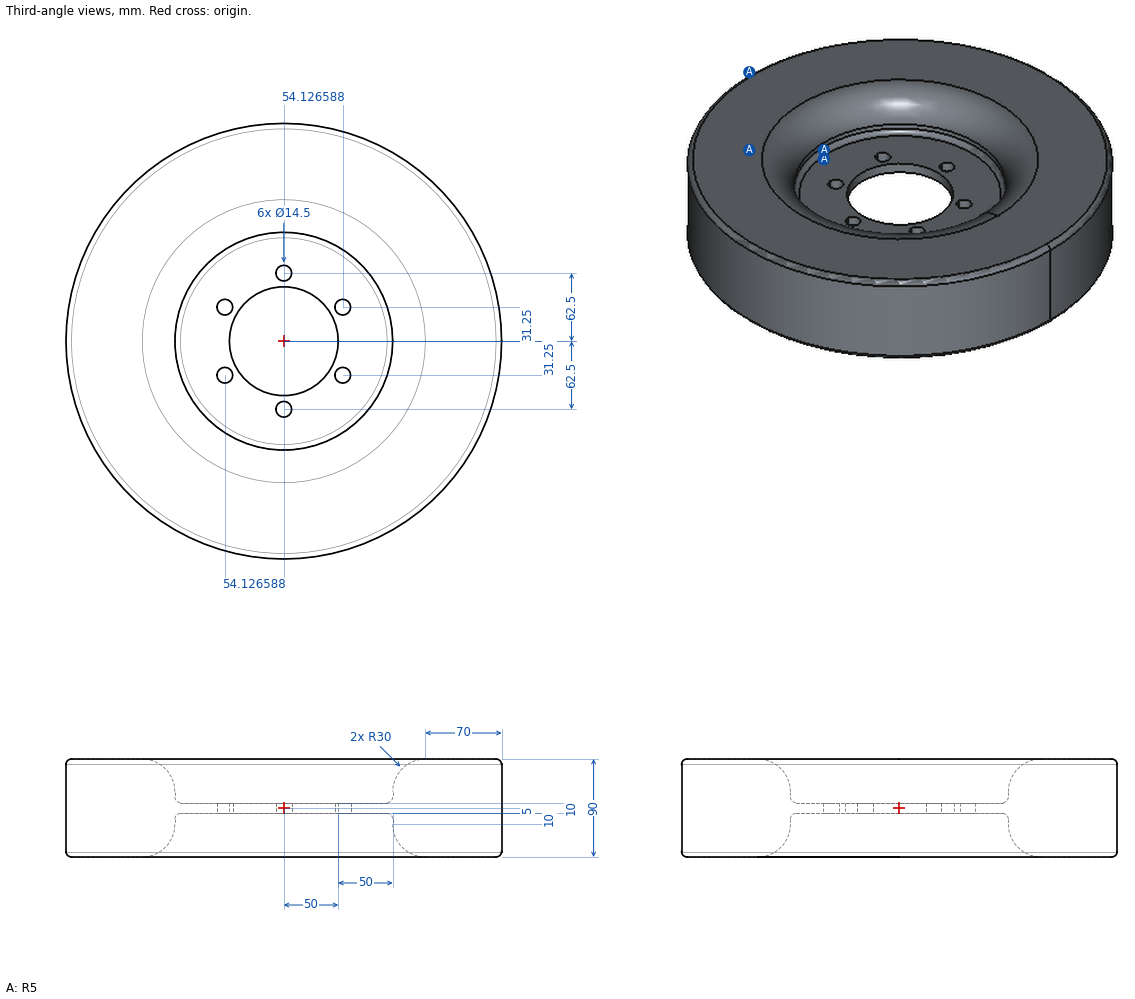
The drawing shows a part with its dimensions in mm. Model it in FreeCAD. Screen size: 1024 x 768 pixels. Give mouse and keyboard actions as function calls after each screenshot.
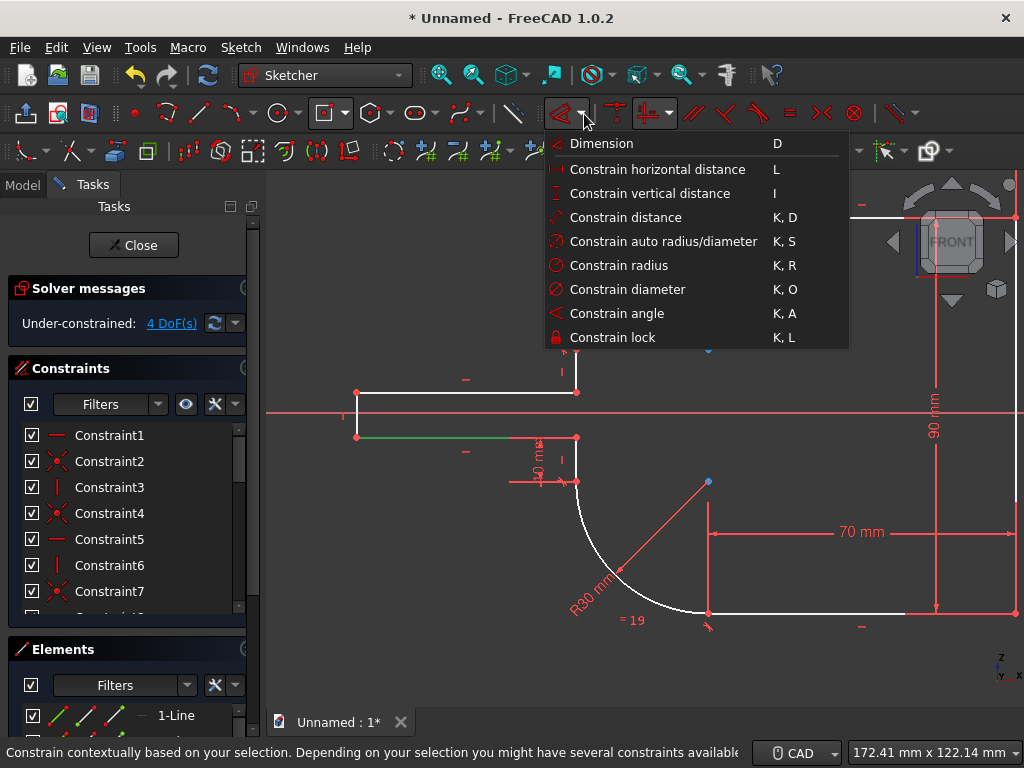
click(697, 169)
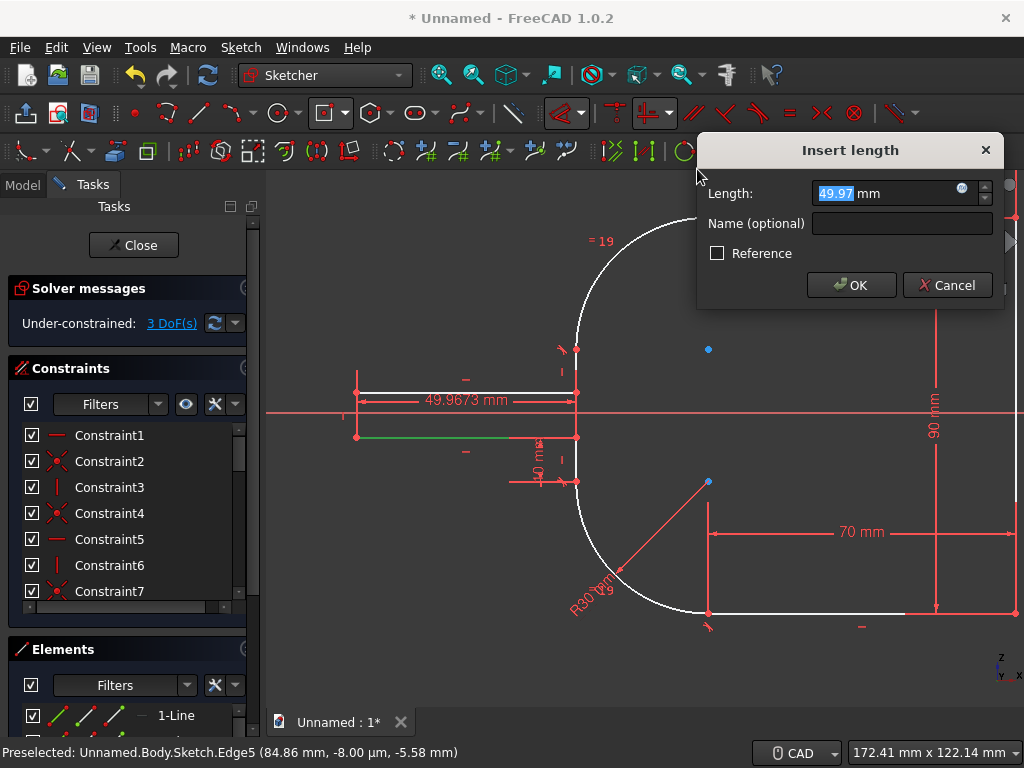
text(50)
key(Return)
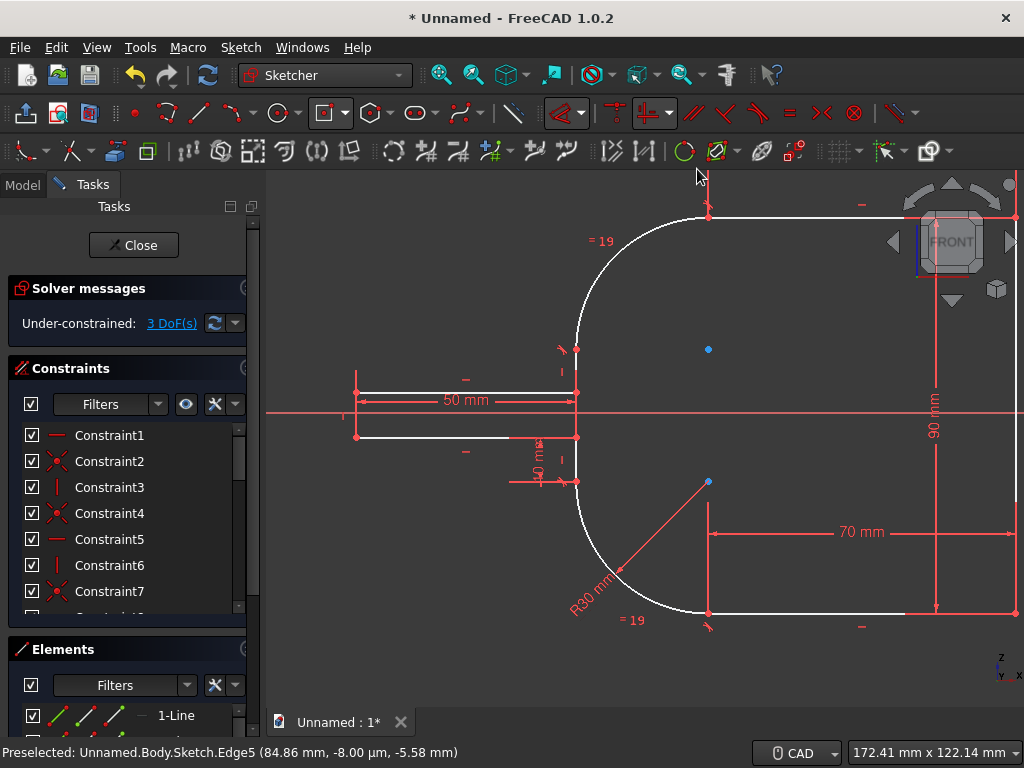
scroll(356, 424, up, 2)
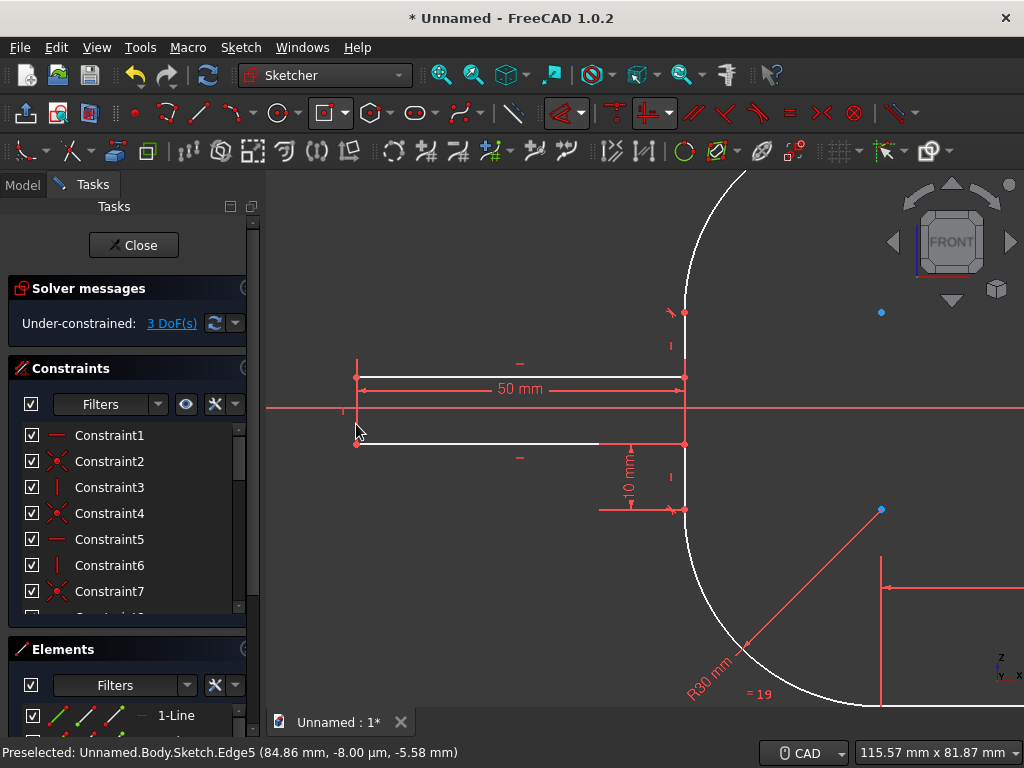
click(357, 424)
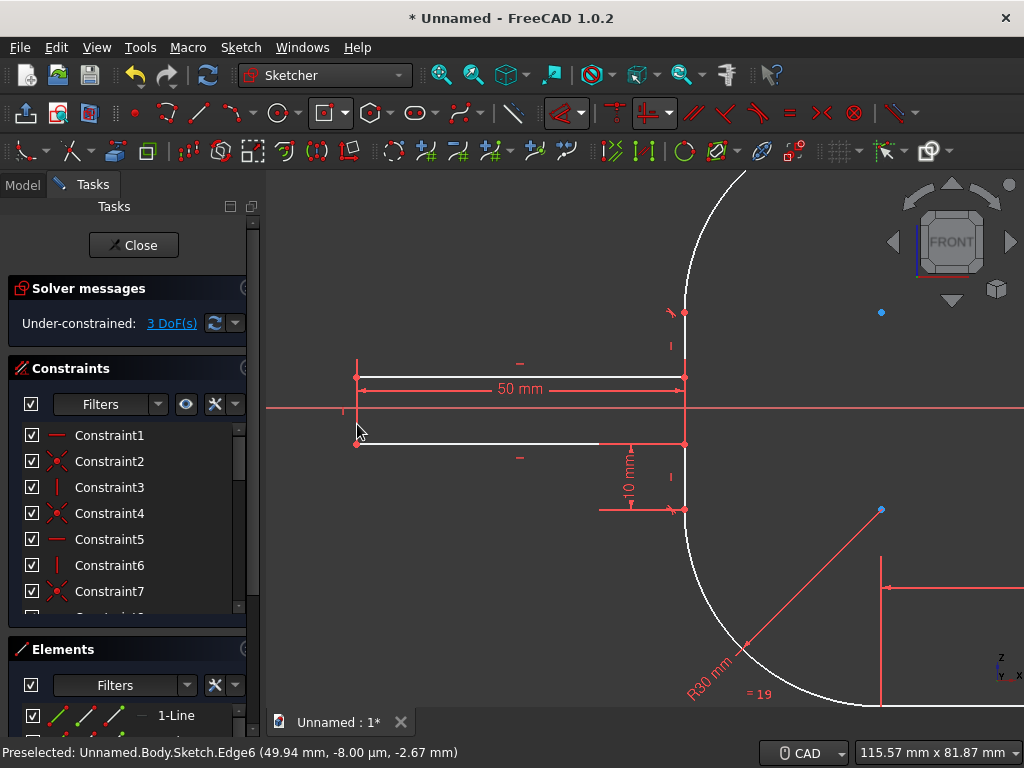
click(584, 114)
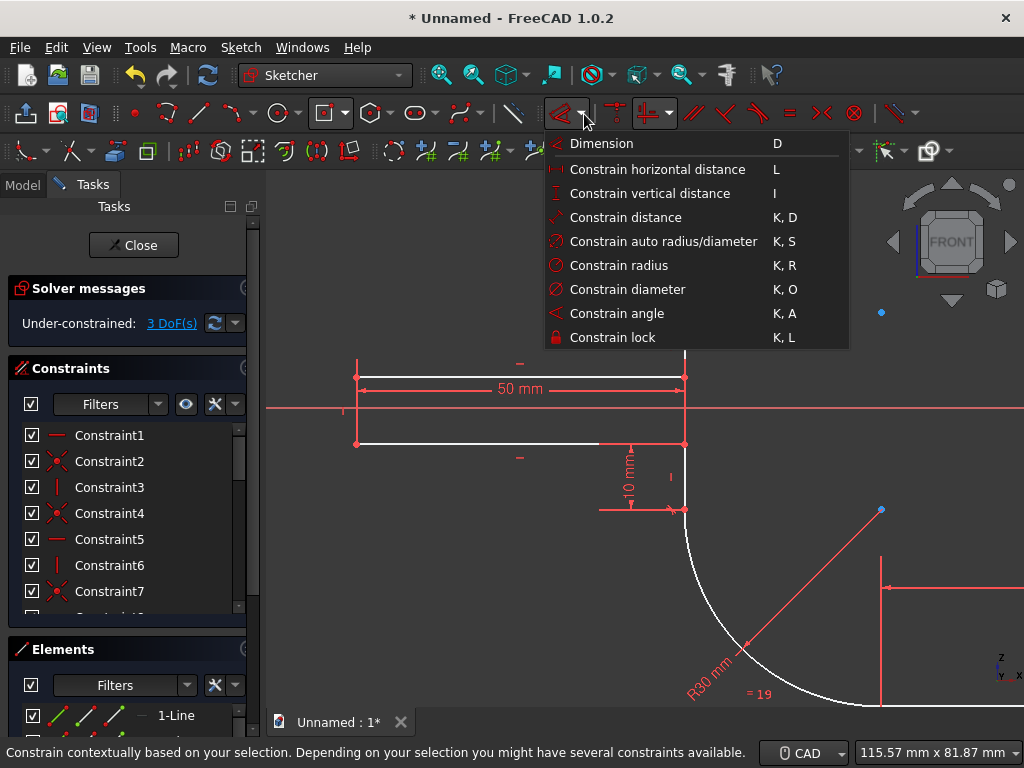
click(697, 193)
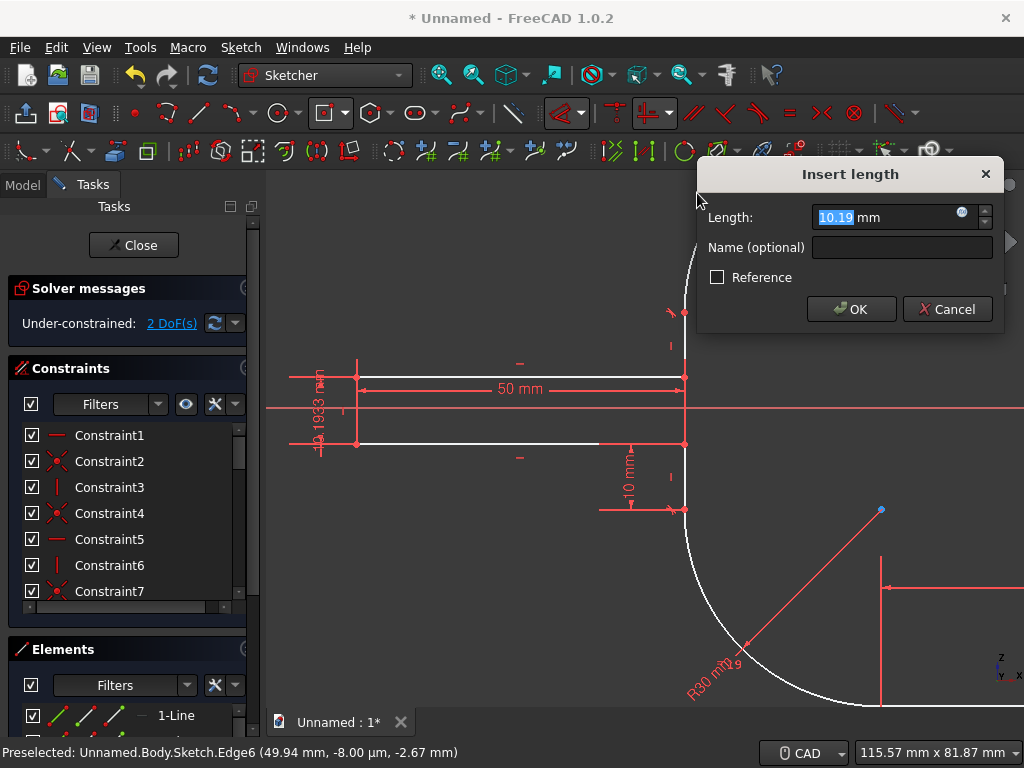
text(10)
key(Return)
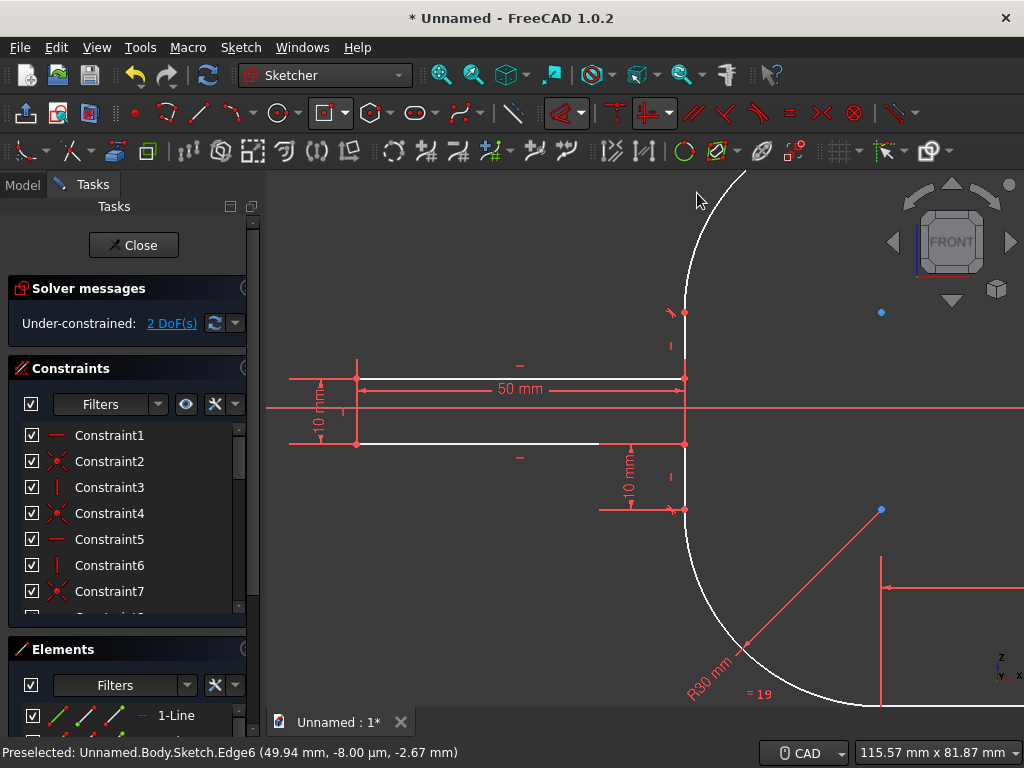
click(685, 444)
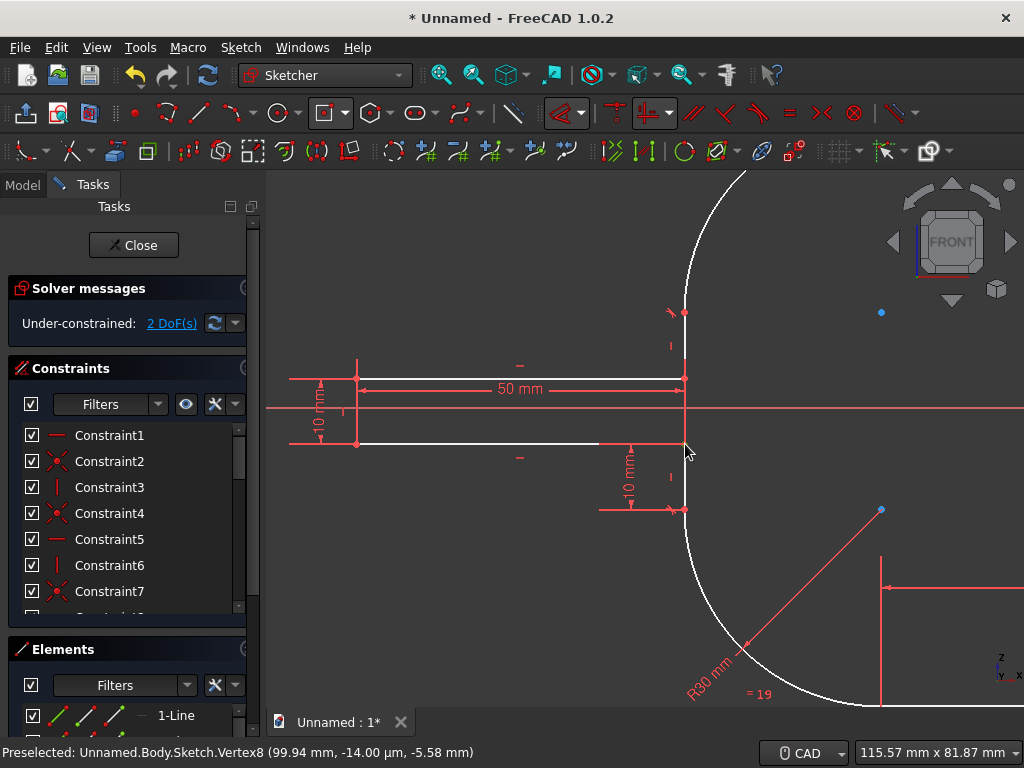
key(i)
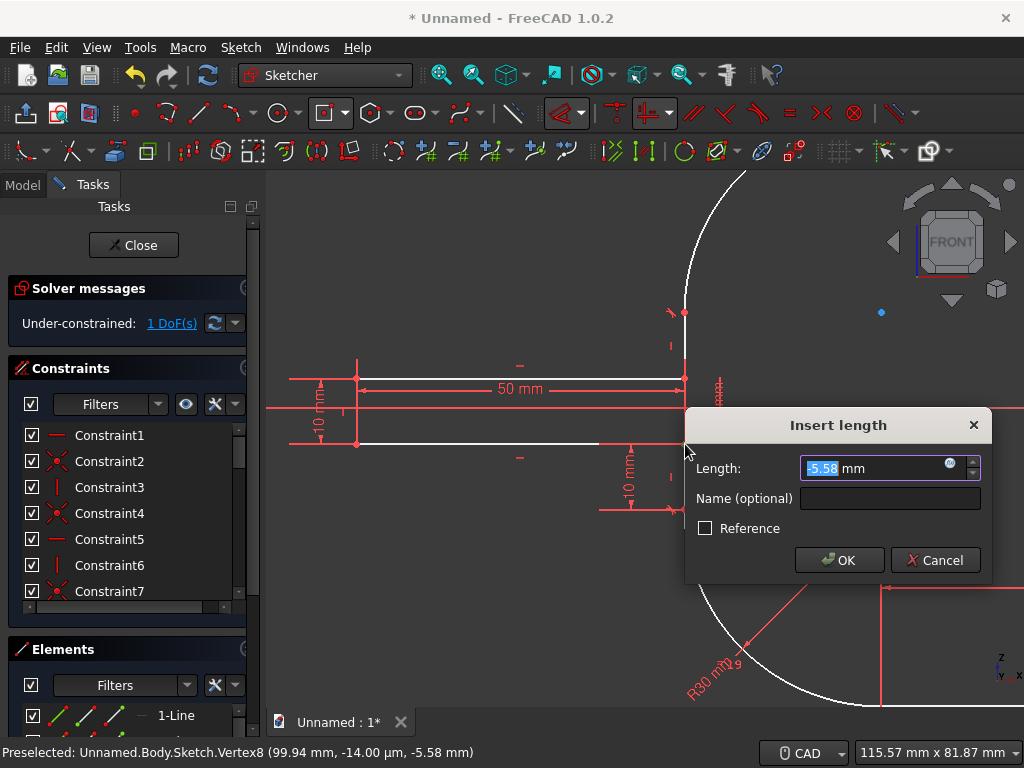
text(-5)
key(Return)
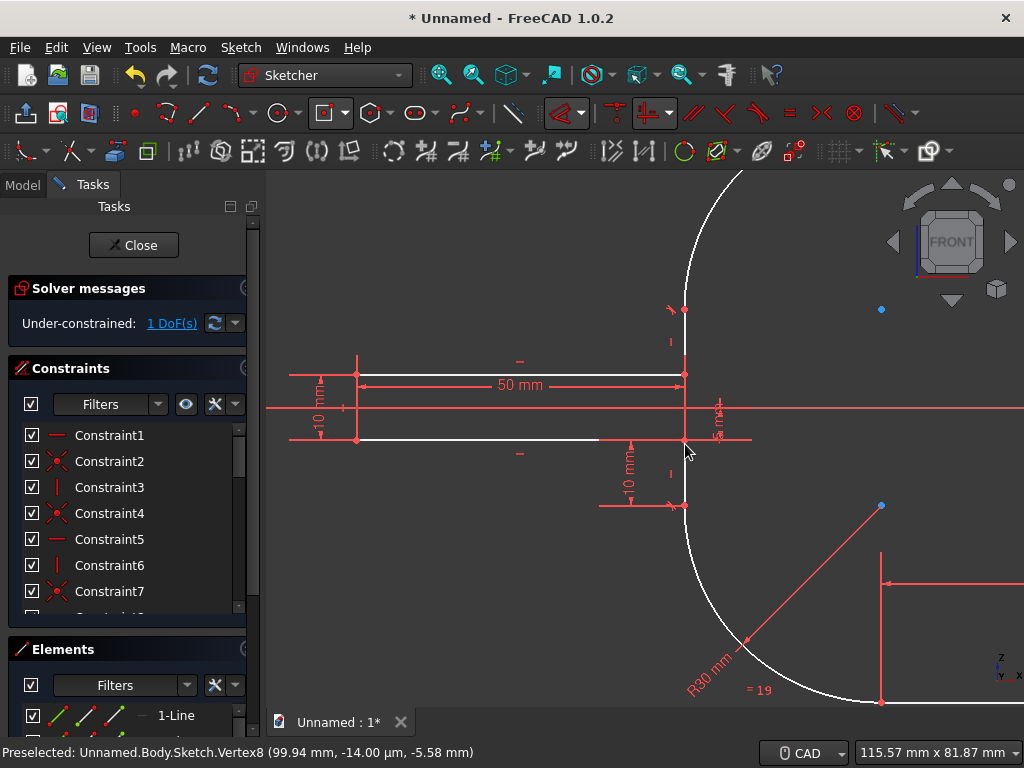
click(357, 440)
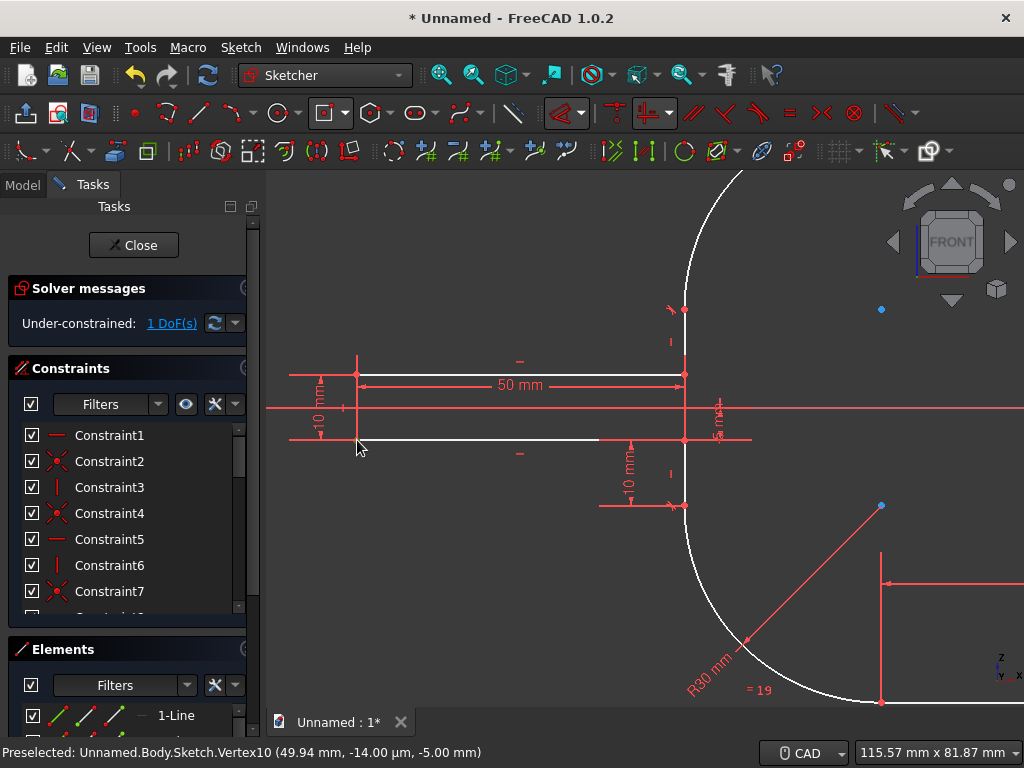
click(584, 114)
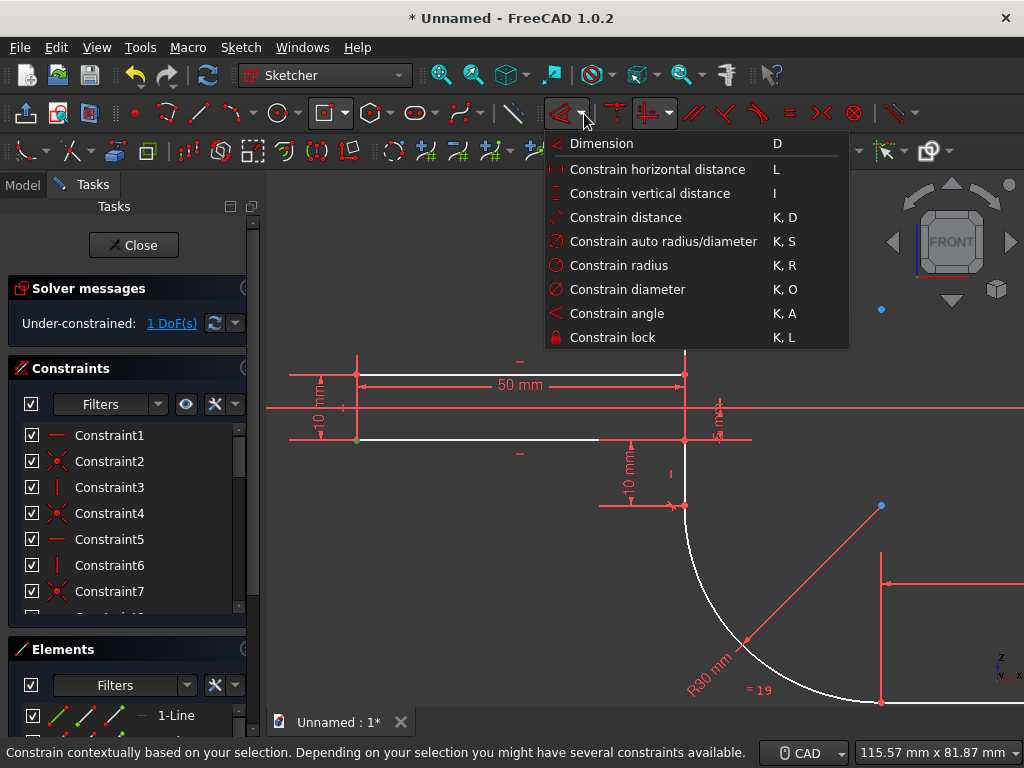
click(697, 169)